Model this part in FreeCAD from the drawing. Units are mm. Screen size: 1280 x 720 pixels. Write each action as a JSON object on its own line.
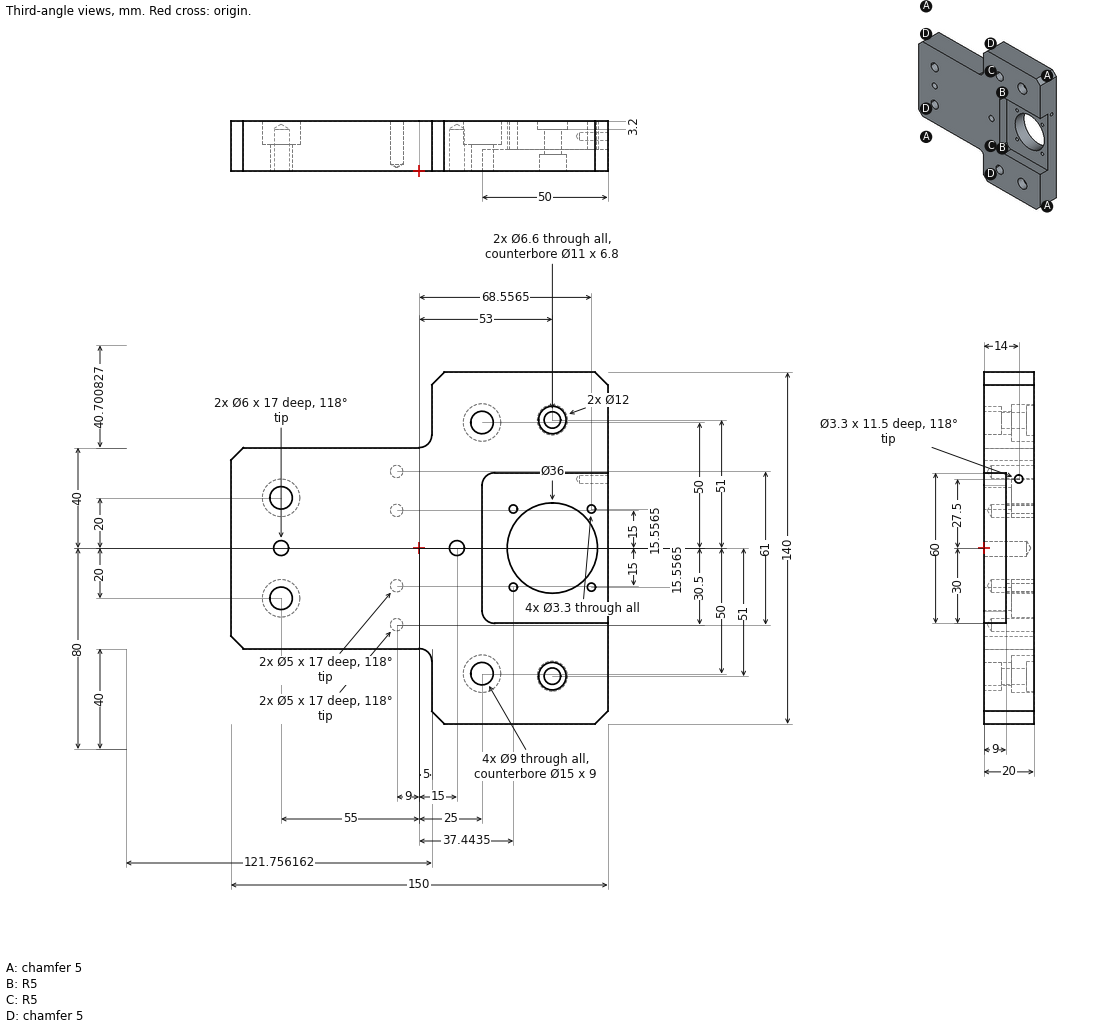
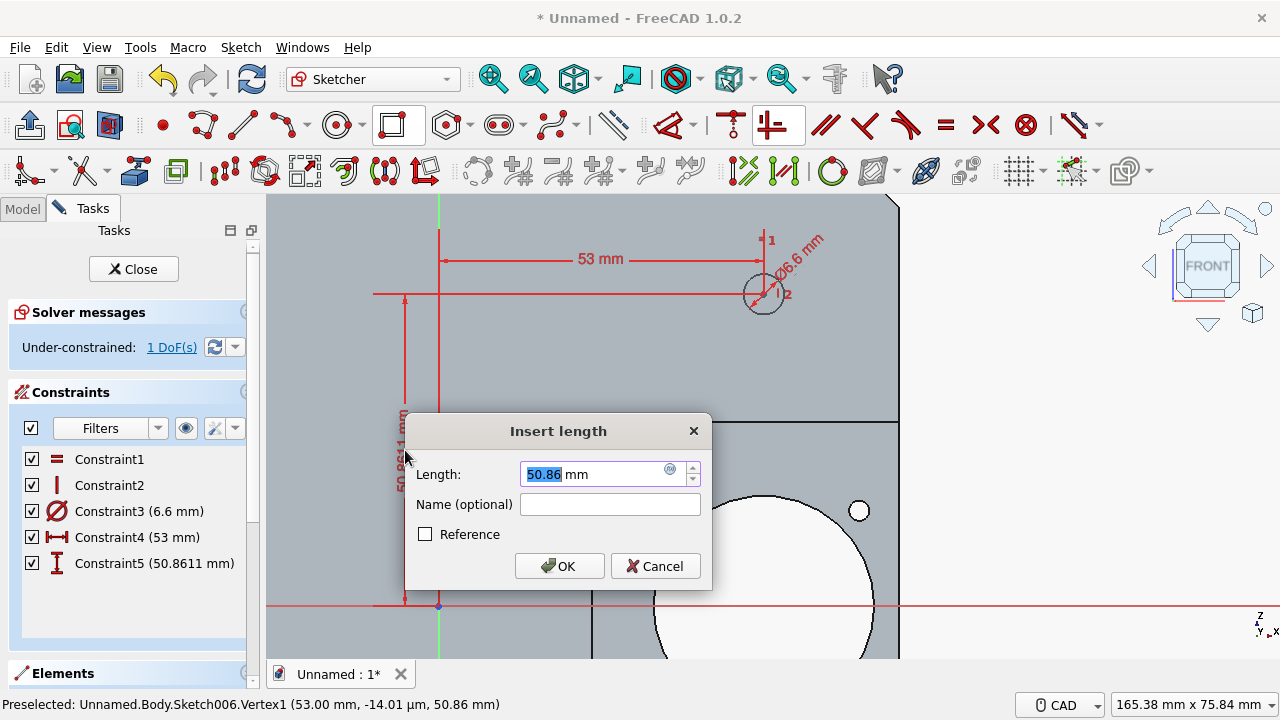
{"action": "type", "text": "51"}
{"action": "key", "text": "Return"}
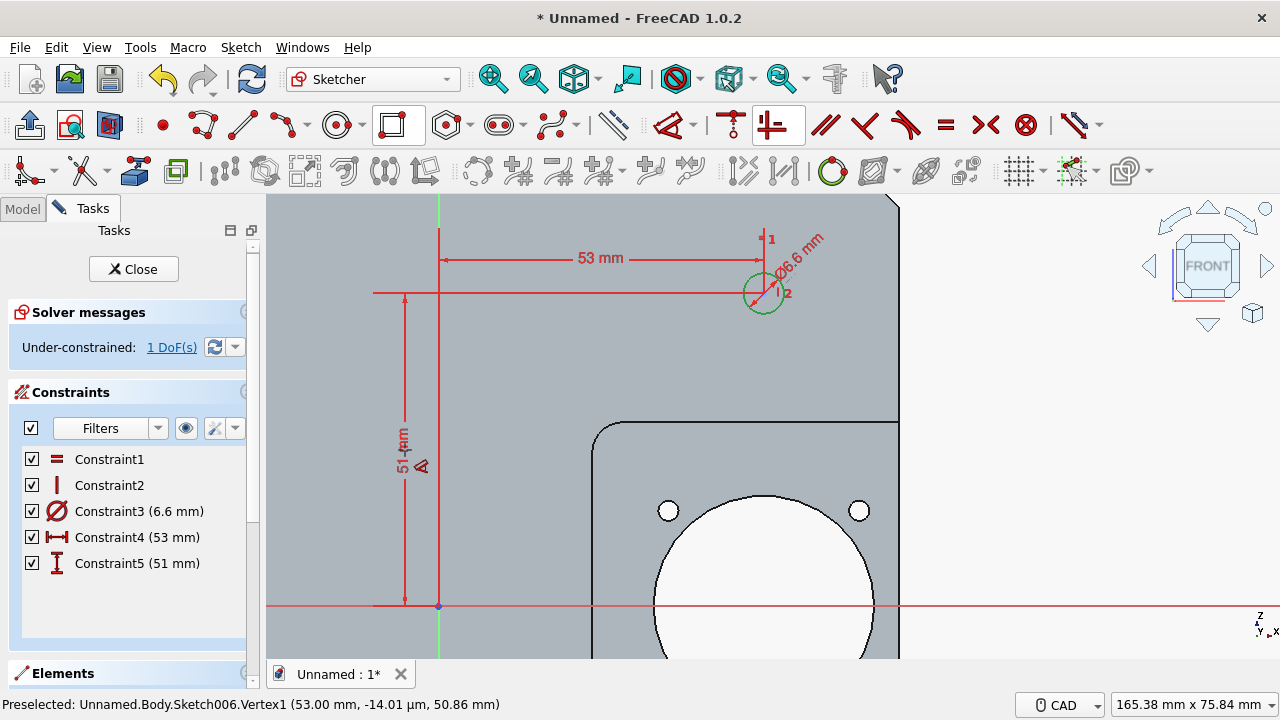
{"action": "scroll", "coordinate": [780, 280], "scroll_direction": "down", "scroll_amount": 4}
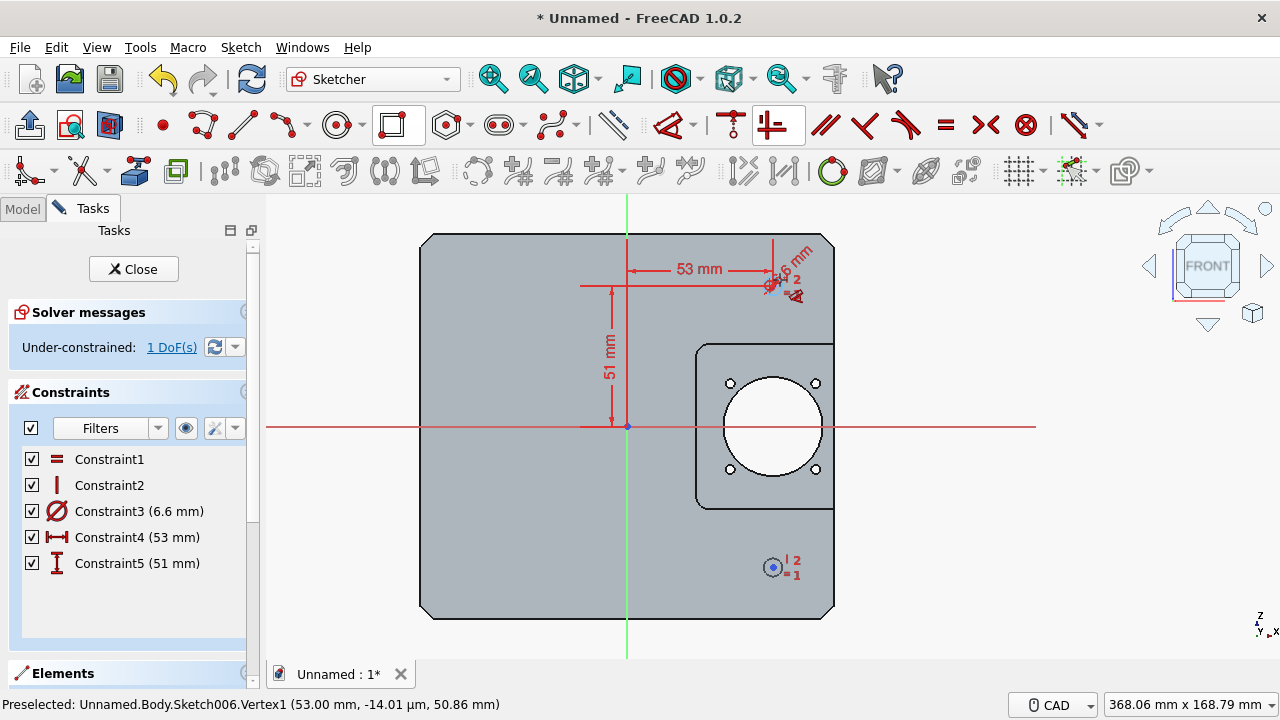
{"action": "left_click", "coordinate": [773, 567]}
{"action": "left_click", "coordinate": [593, 497]}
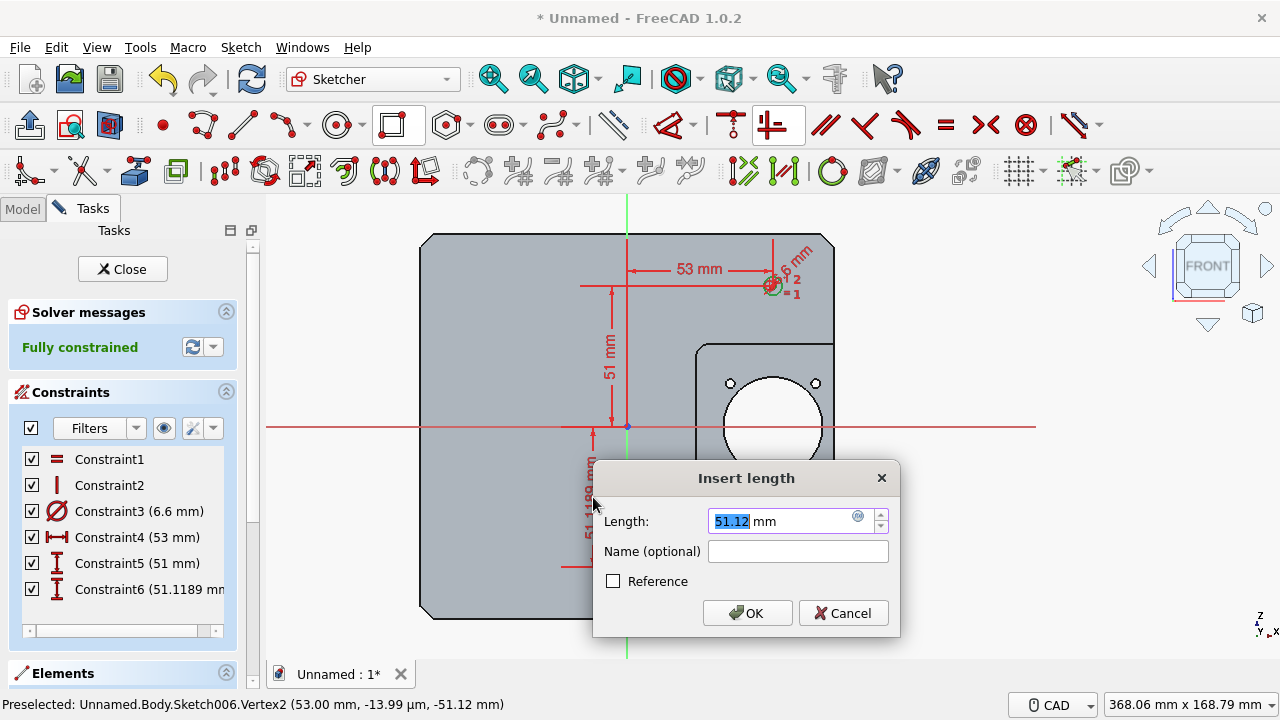
{"action": "type", "text": "51"}
{"action": "key", "text": "Return"}
{"action": "key", "text": "Escape"}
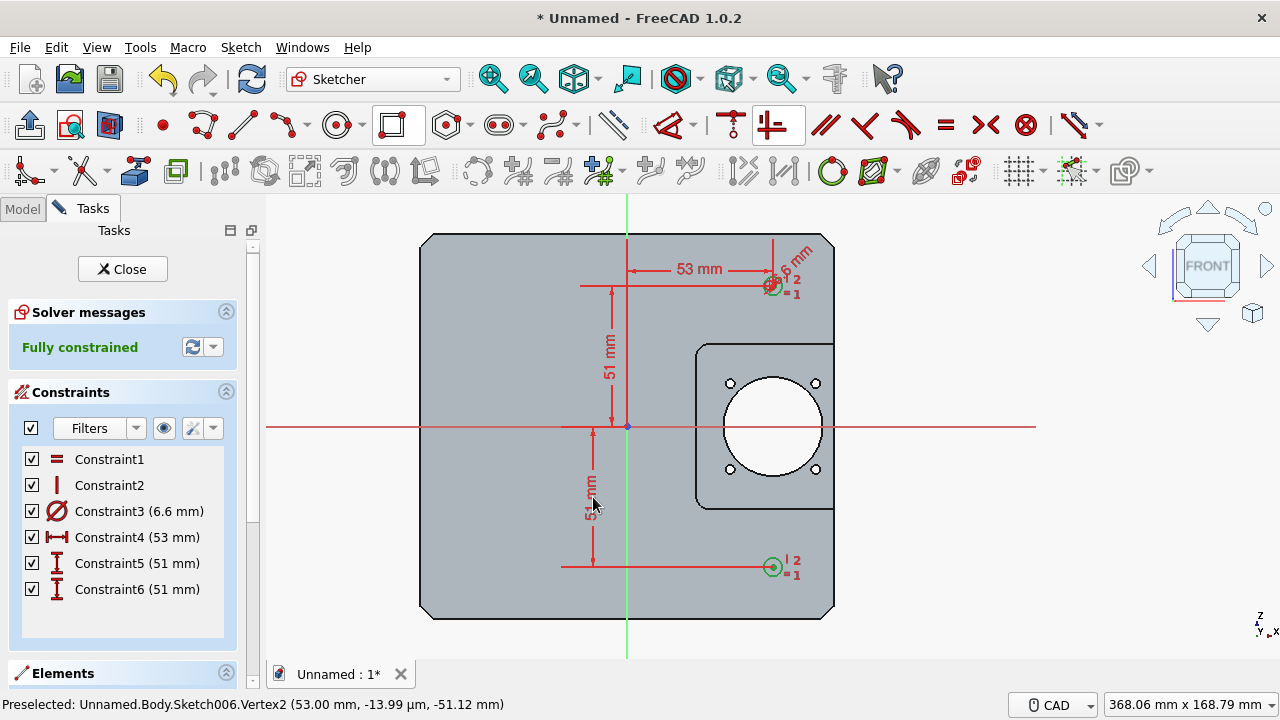
{"action": "left_click", "coordinate": [123, 269]}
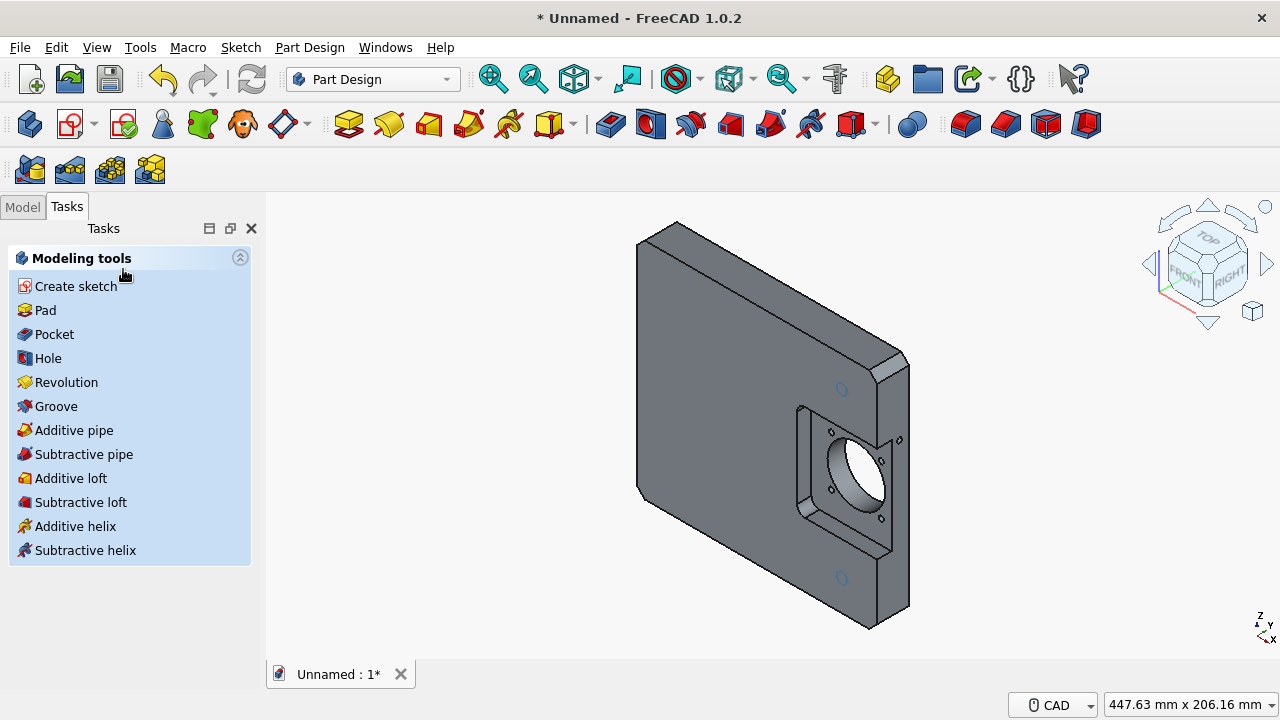
{"action": "left_click", "coordinate": [652, 124]}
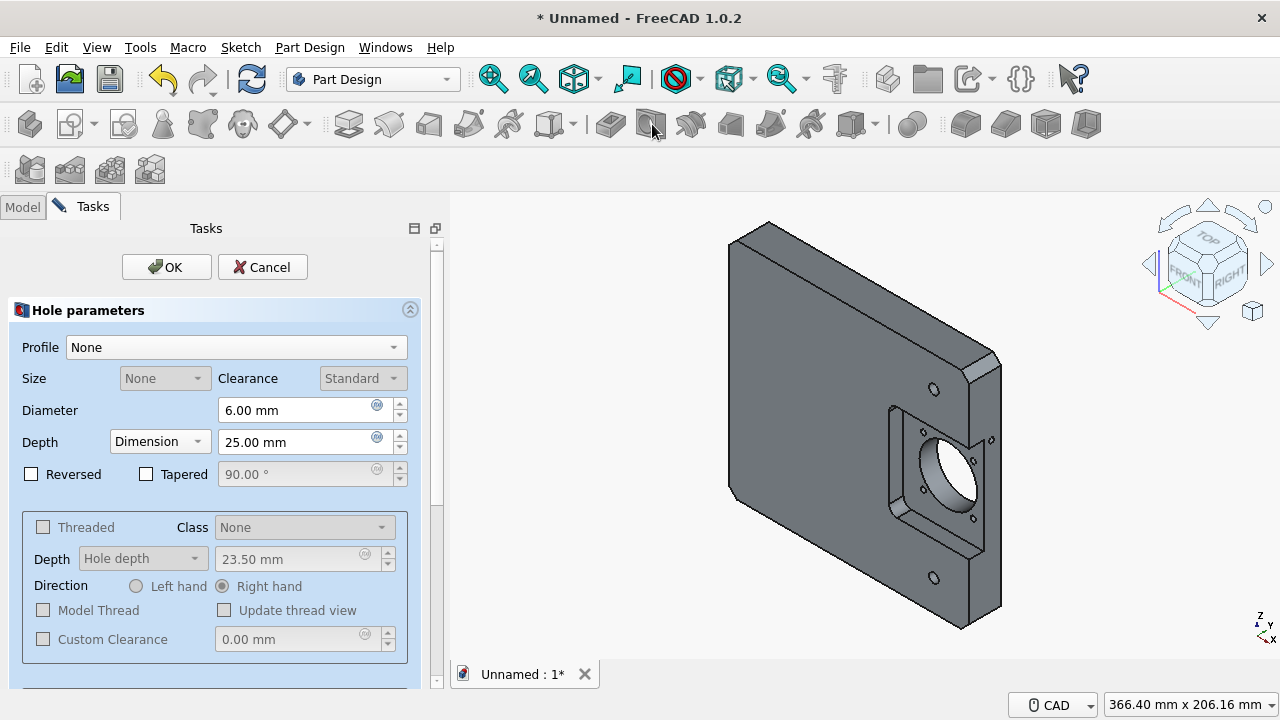
{"action": "triple_click", "coordinate": [305, 410]}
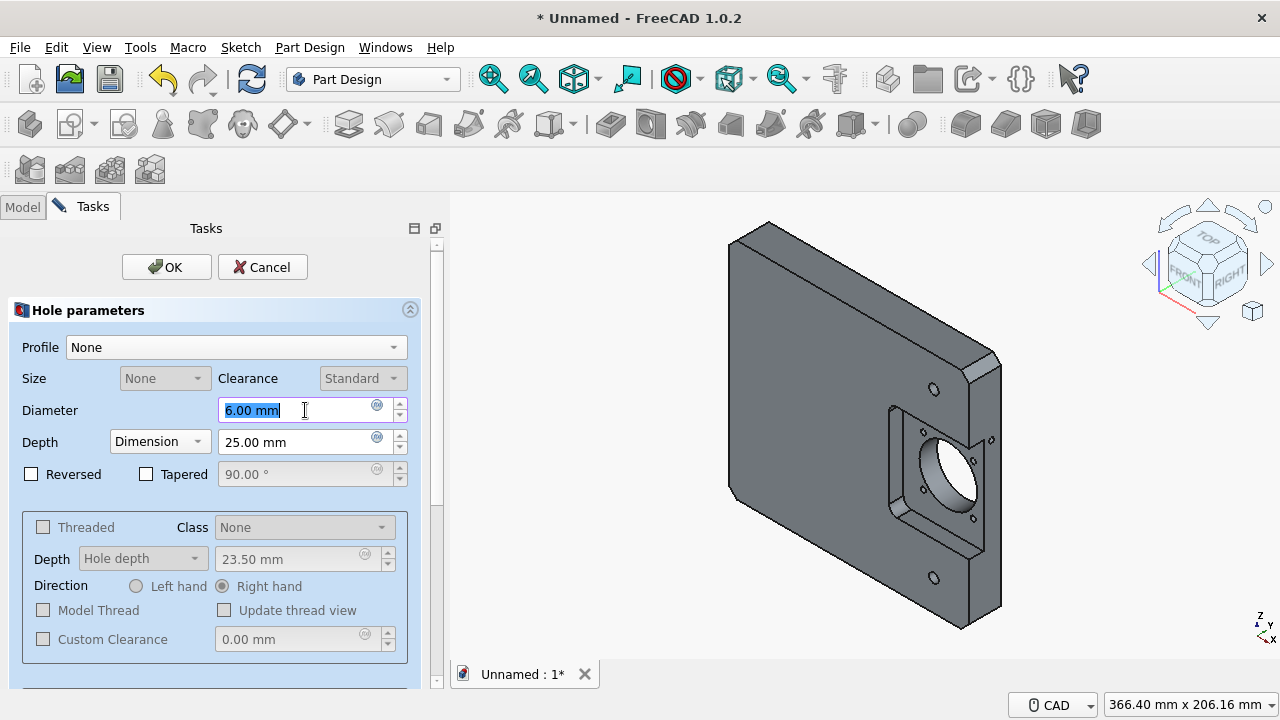
{"action": "type", "text": "6.6"}
{"action": "key", "text": "Tab"}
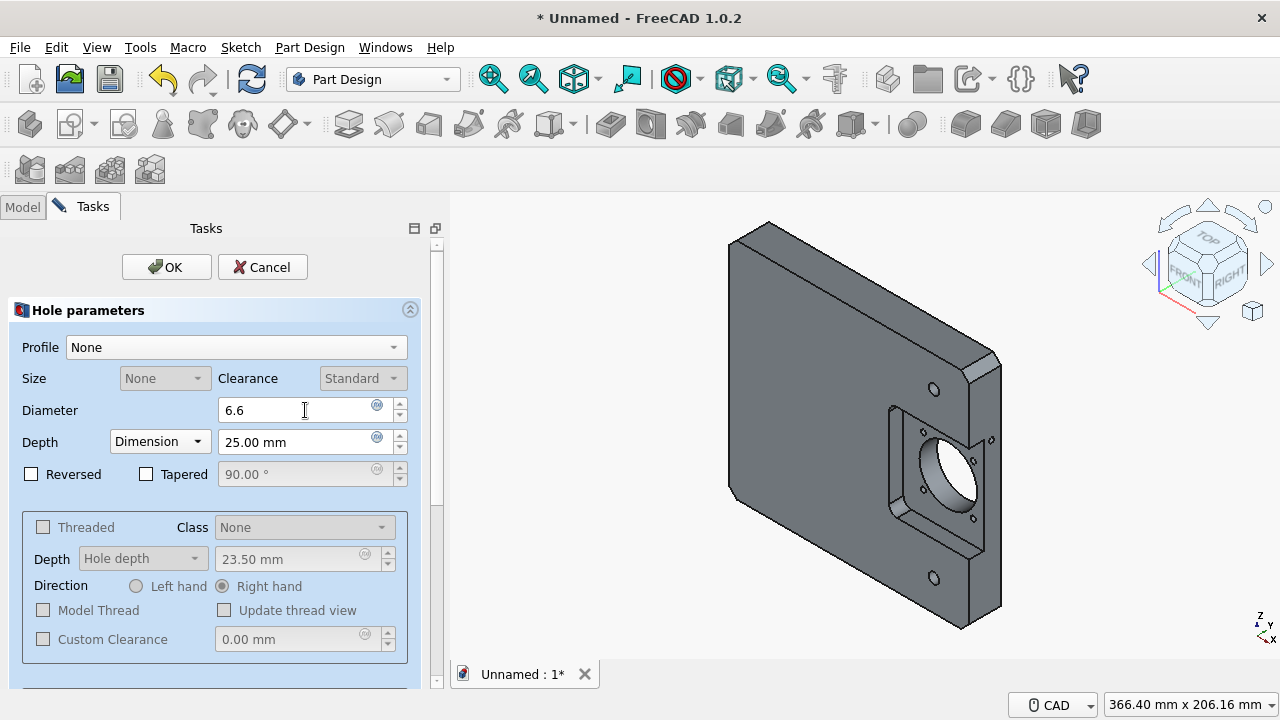
{"action": "left_click", "coordinate": [161, 442]}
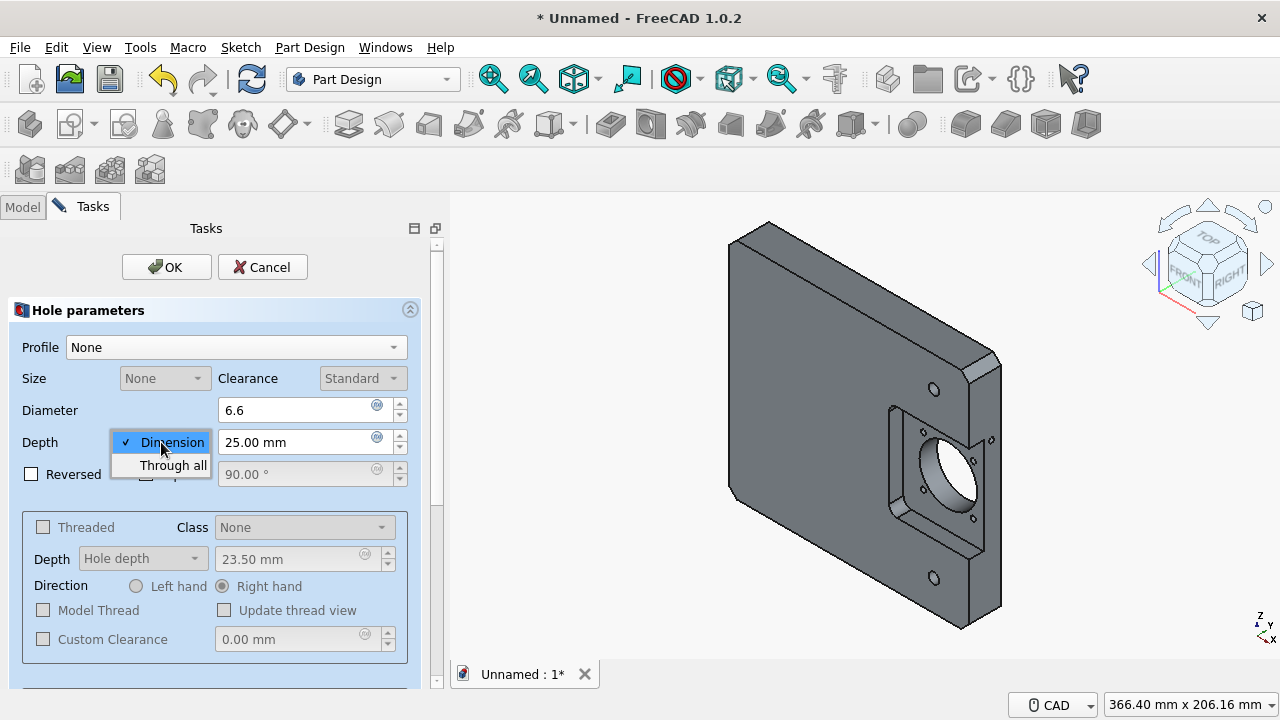
{"action": "left_click", "coordinate": [160, 466]}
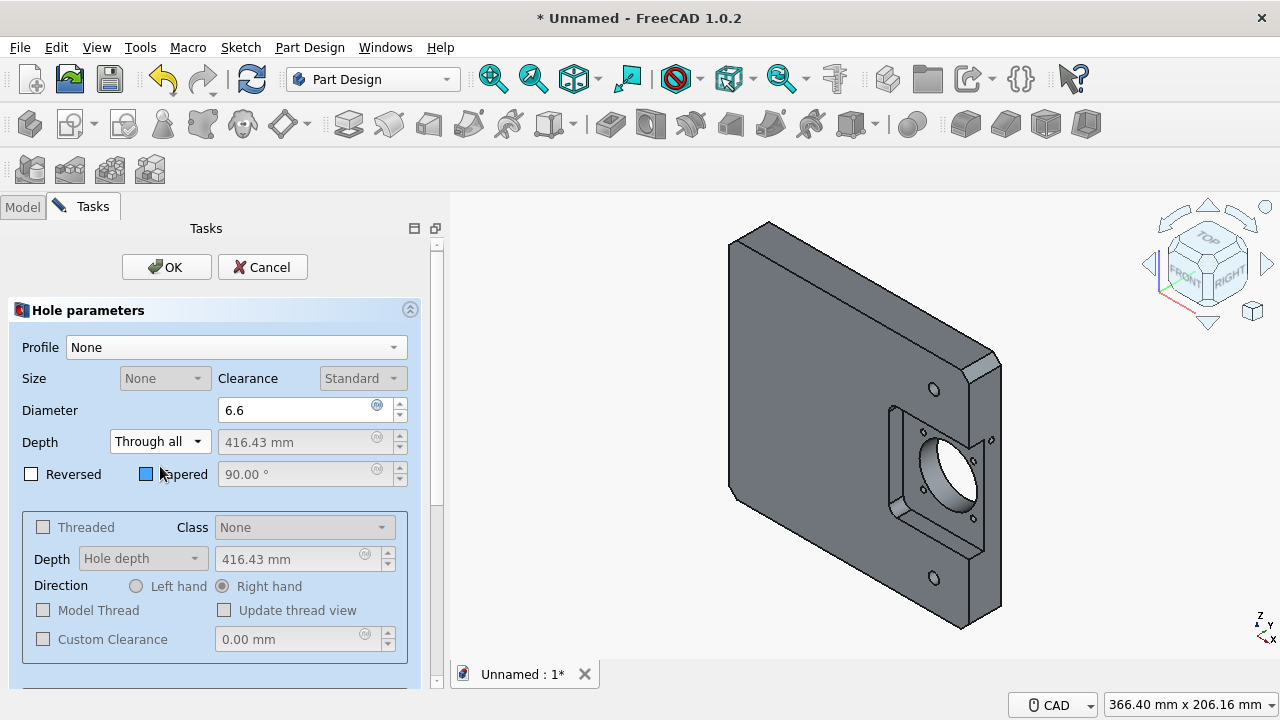
{"action": "scroll", "coordinate": [437, 463], "scroll_direction": "down", "scroll_amount": 2}